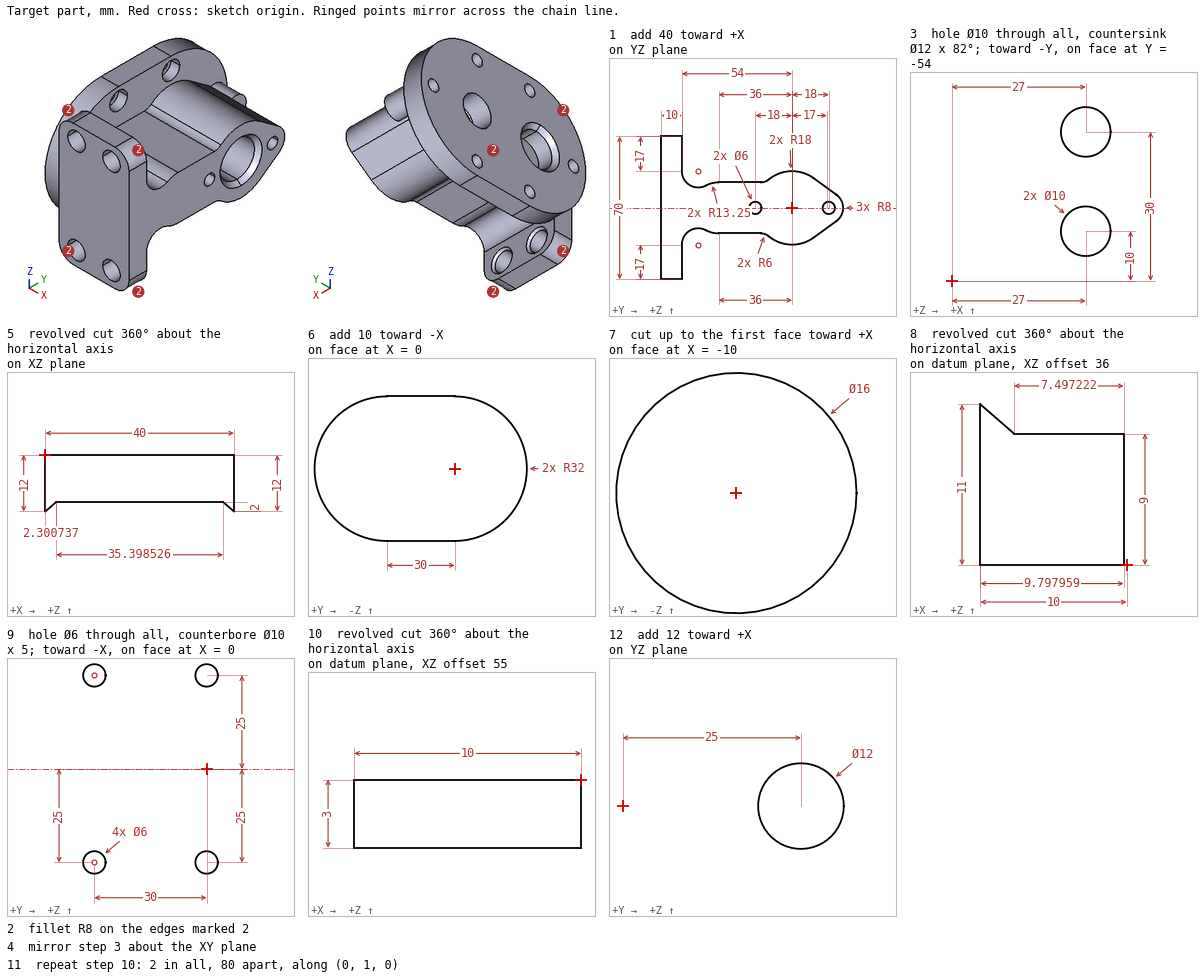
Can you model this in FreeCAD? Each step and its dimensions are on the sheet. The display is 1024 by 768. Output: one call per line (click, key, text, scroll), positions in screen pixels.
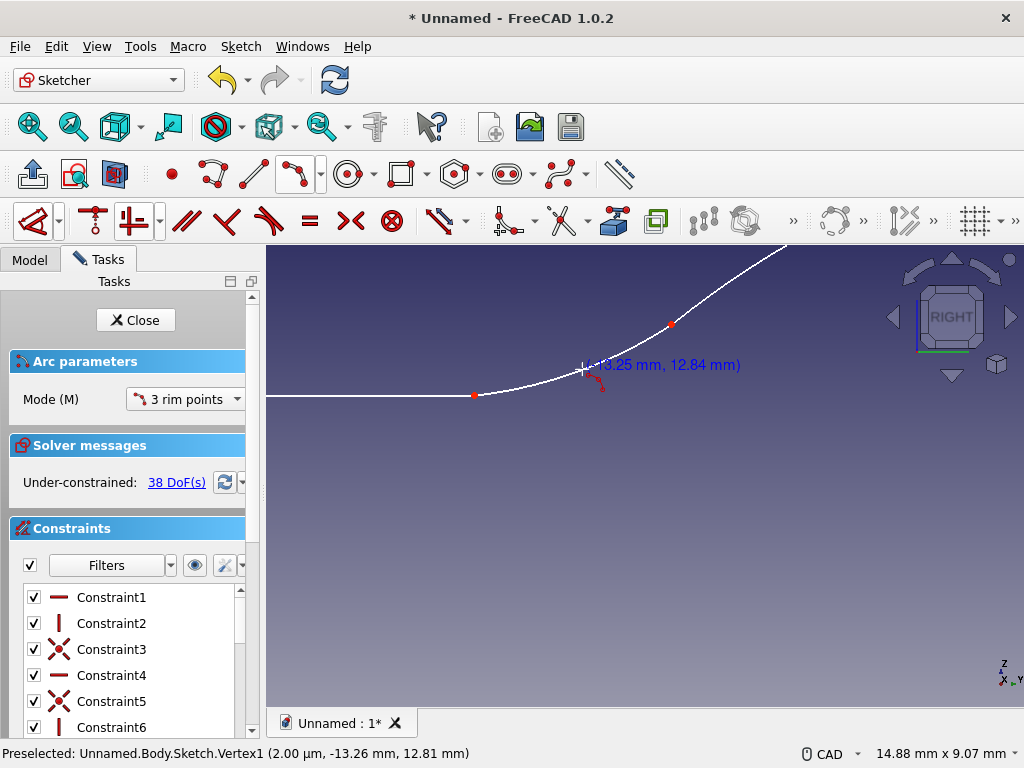
click(348, 174)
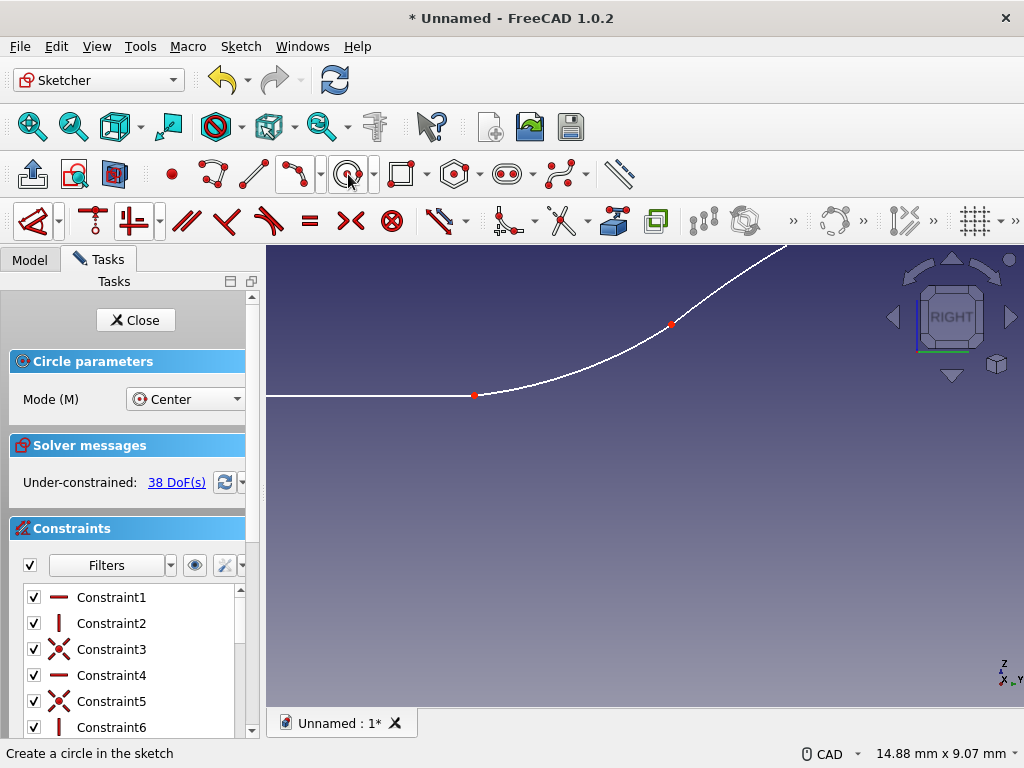
scroll(602, 432, down, 13)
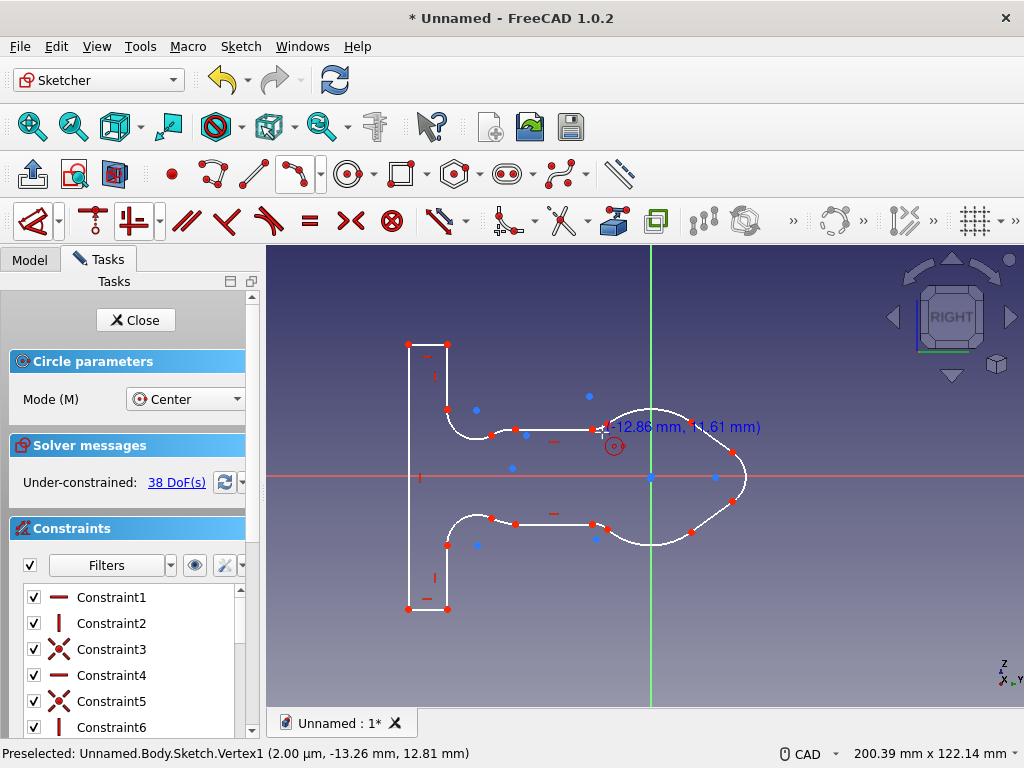
scroll(583, 476, up, 4)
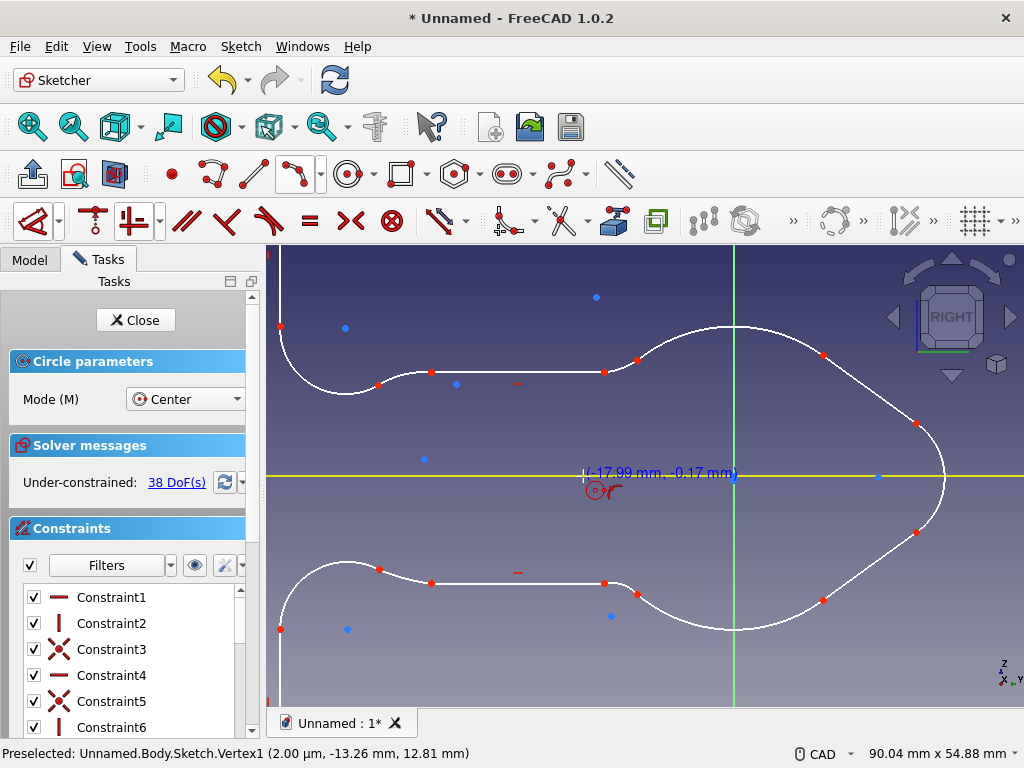
click(582, 476)
click(600, 458)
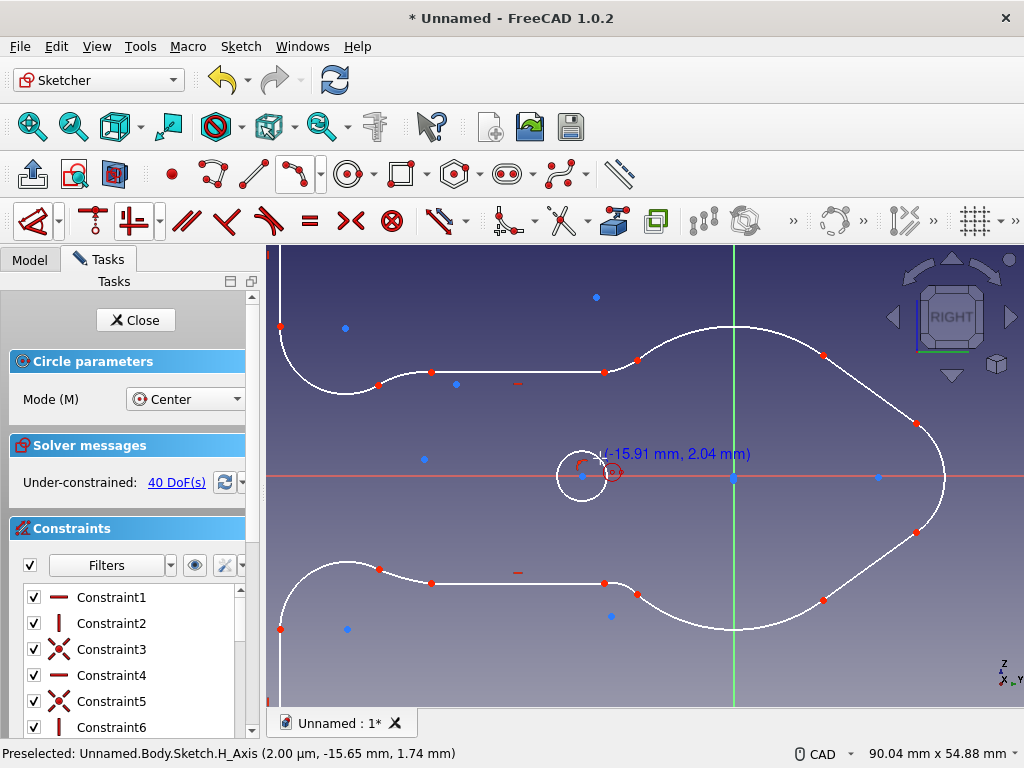
scroll(582, 476, down, 4)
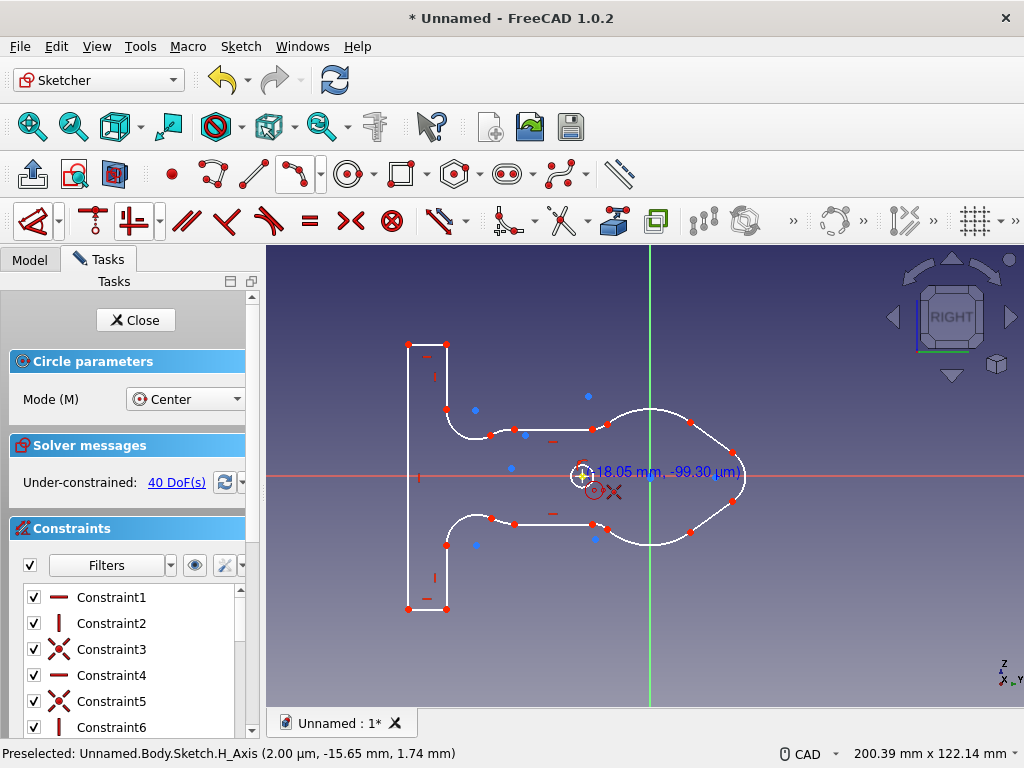
scroll(719, 476, up, 8)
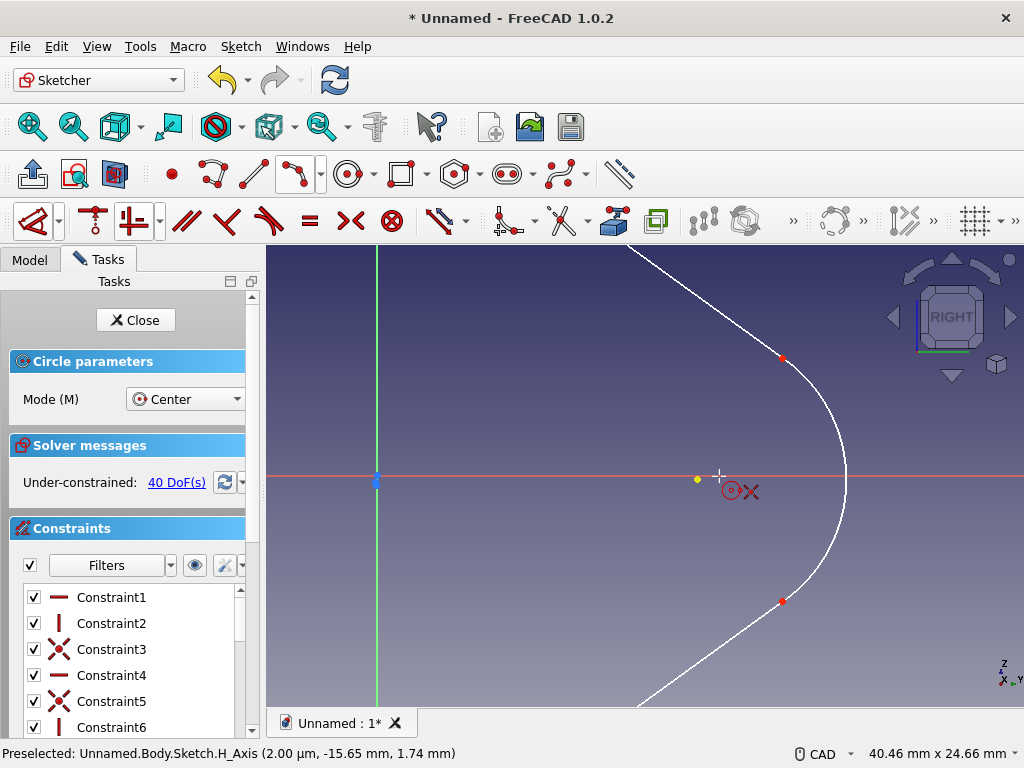
click(715, 476)
click(754, 436)
key(Escape)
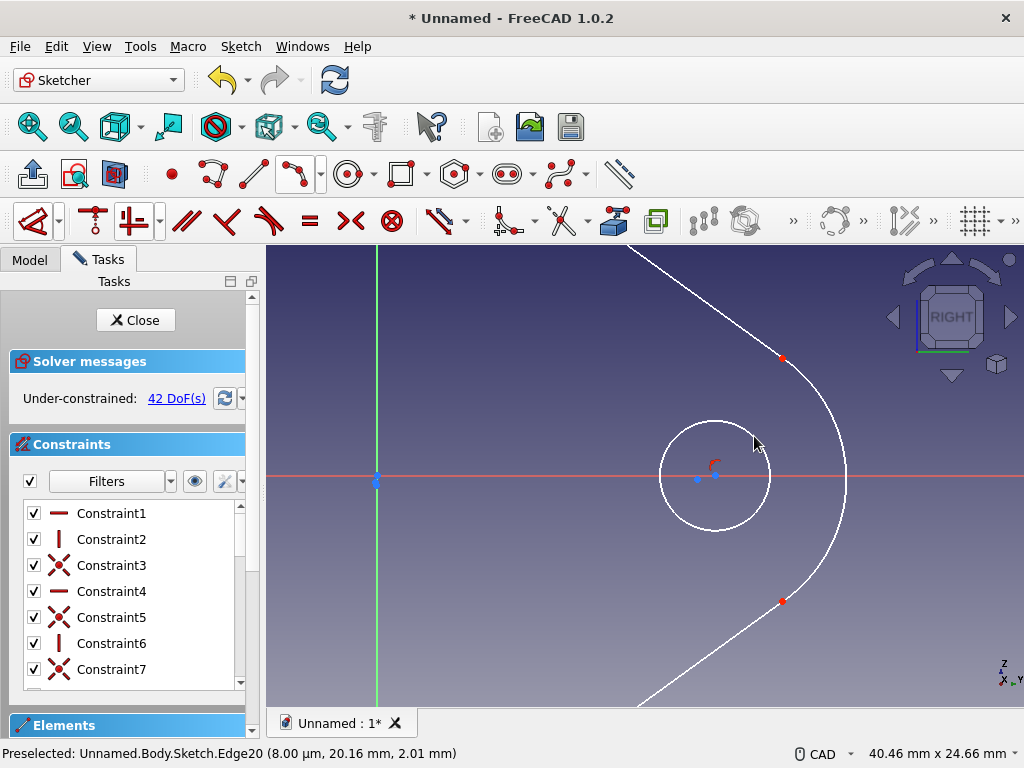
scroll(719, 476, down, 8)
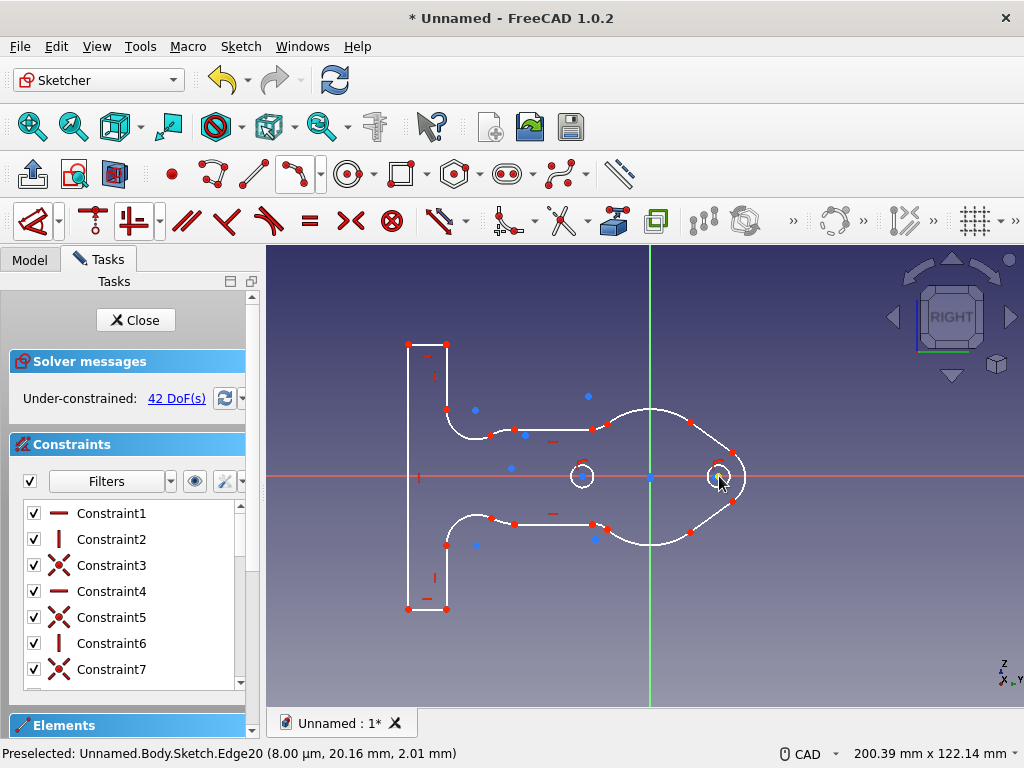
click(569, 430)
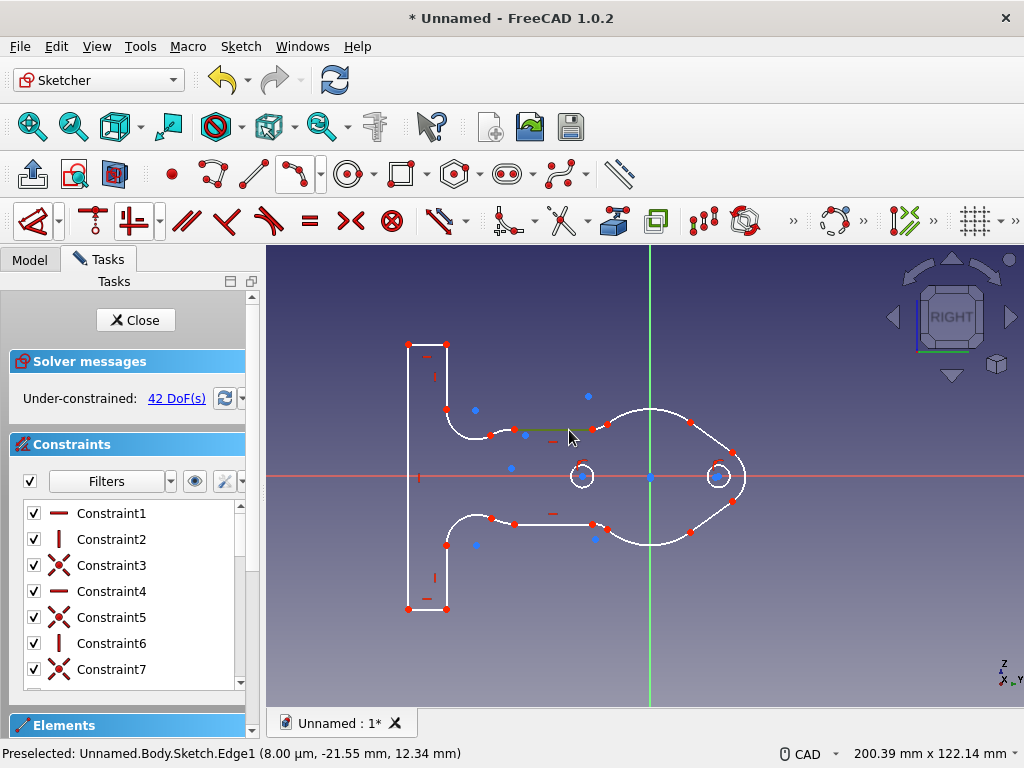
click(502, 431)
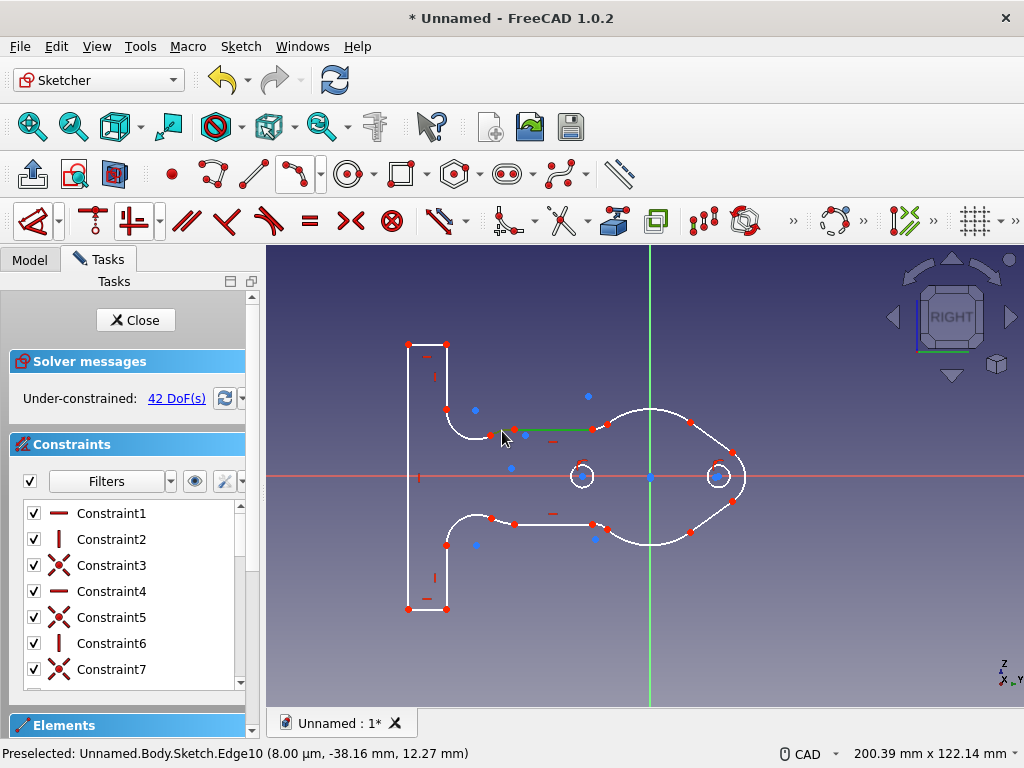
click(269, 222)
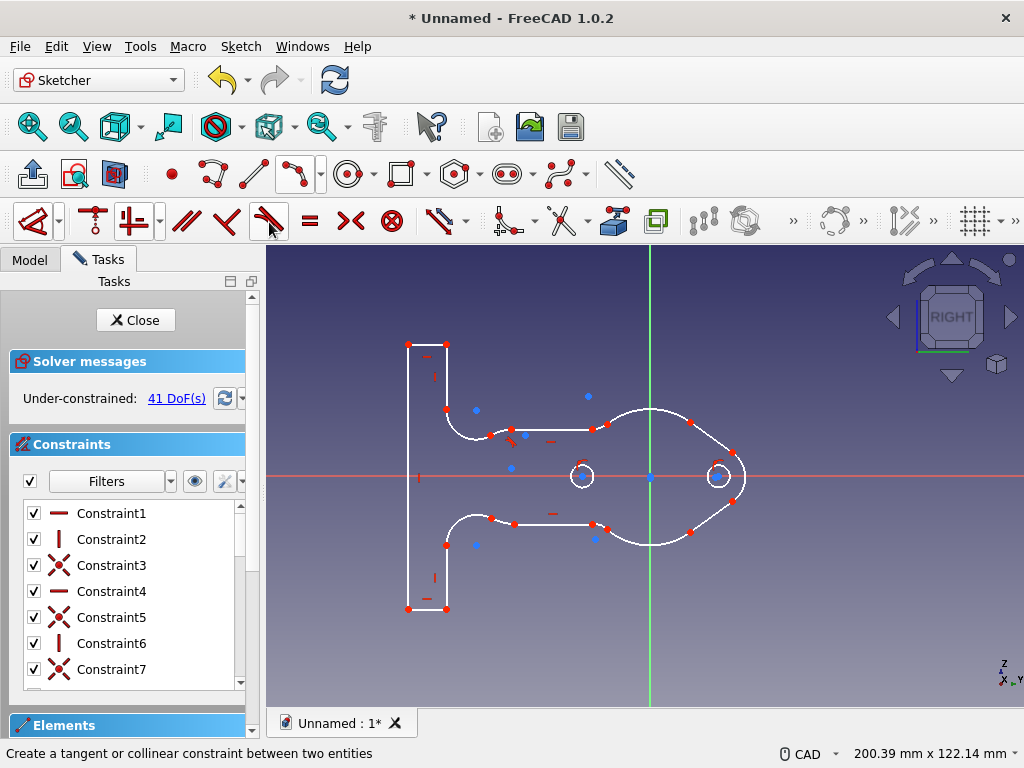
click(568, 430)